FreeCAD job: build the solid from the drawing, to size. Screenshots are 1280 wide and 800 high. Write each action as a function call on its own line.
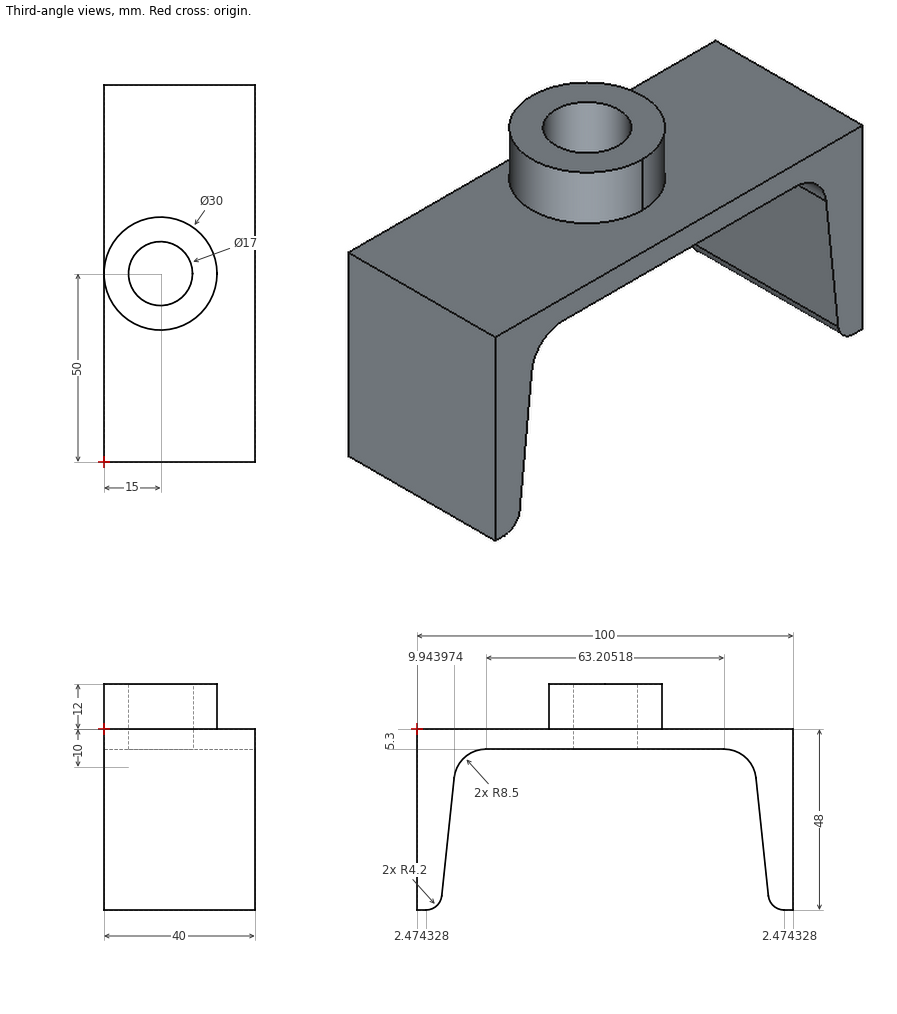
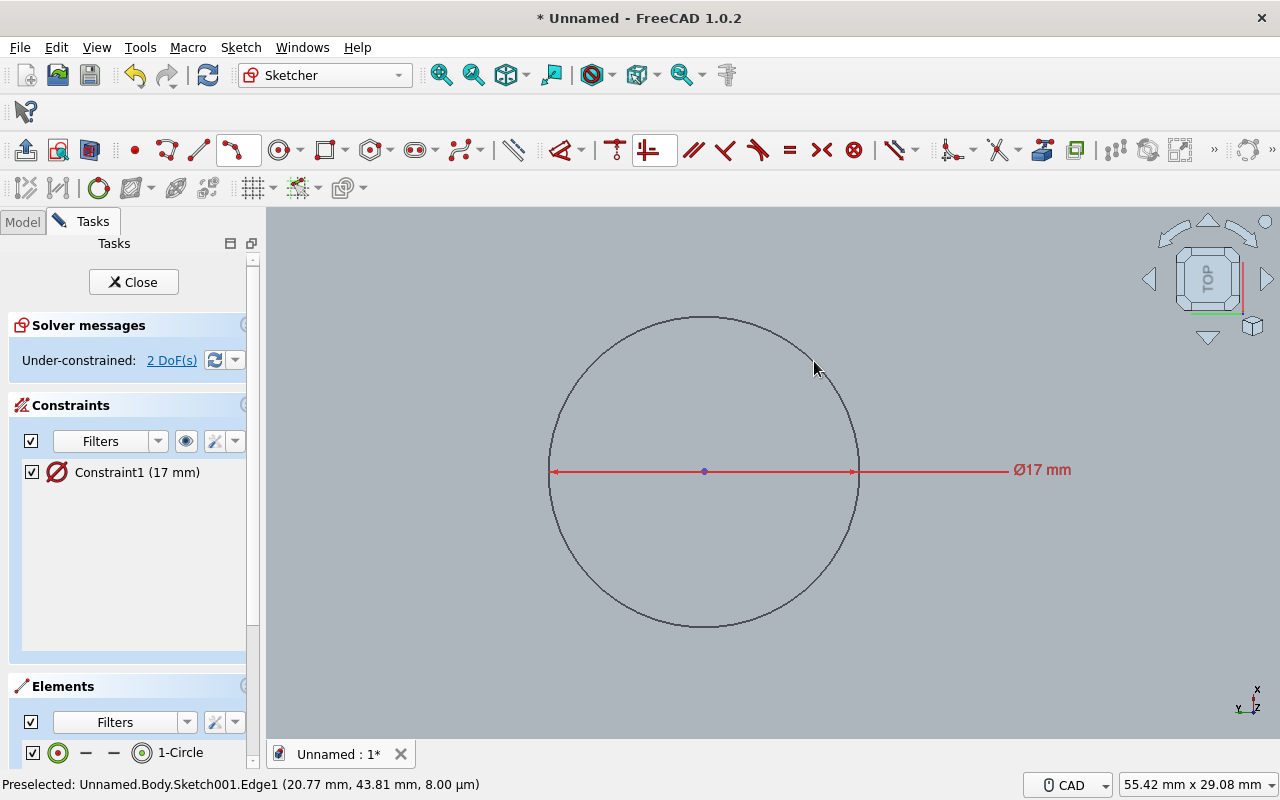
click(560, 150)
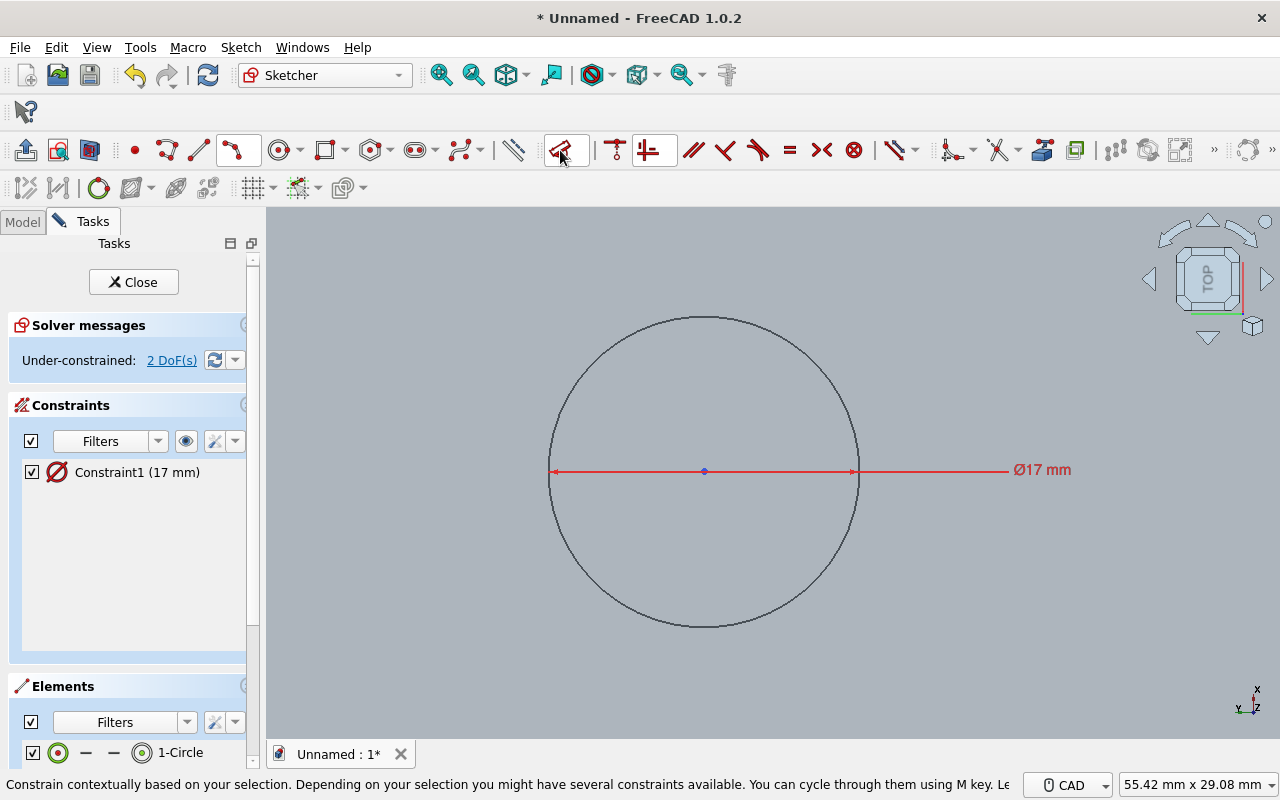
click(704, 472)
click(909, 438)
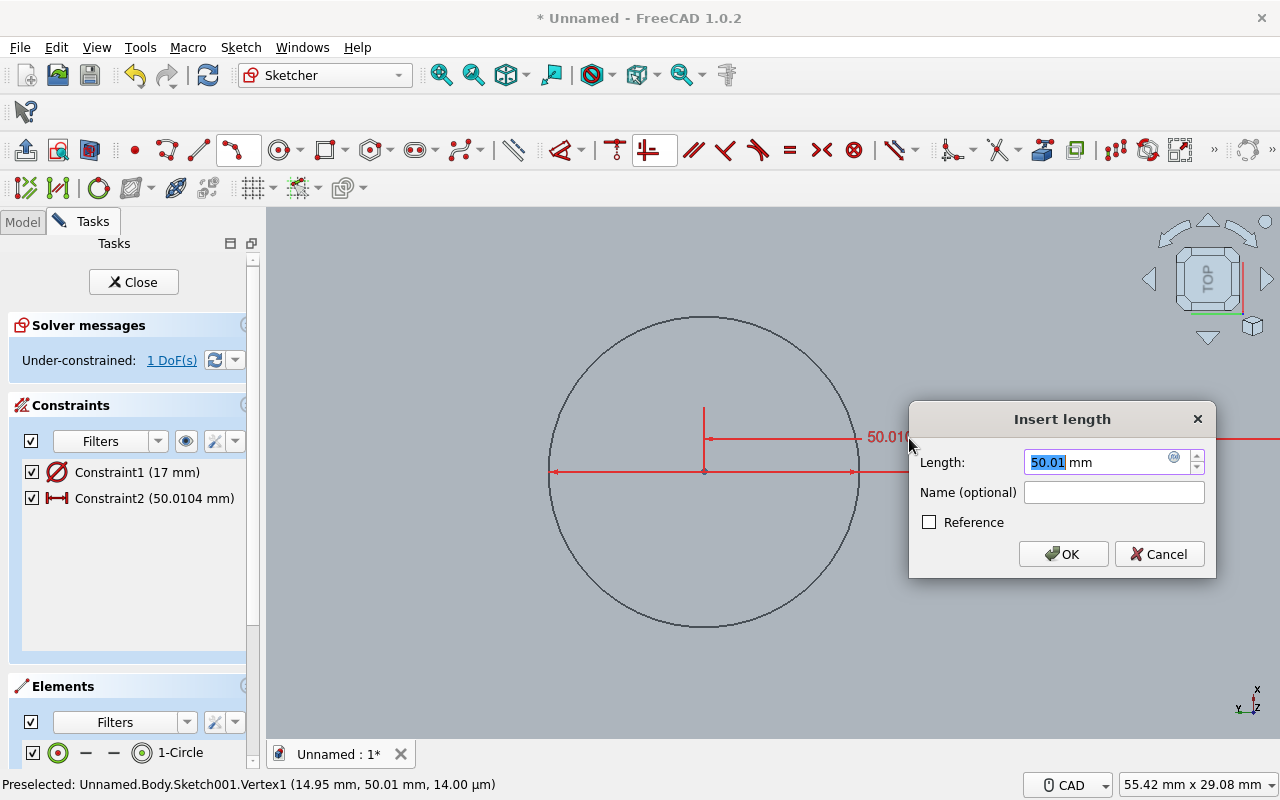
text(50)
key(Return)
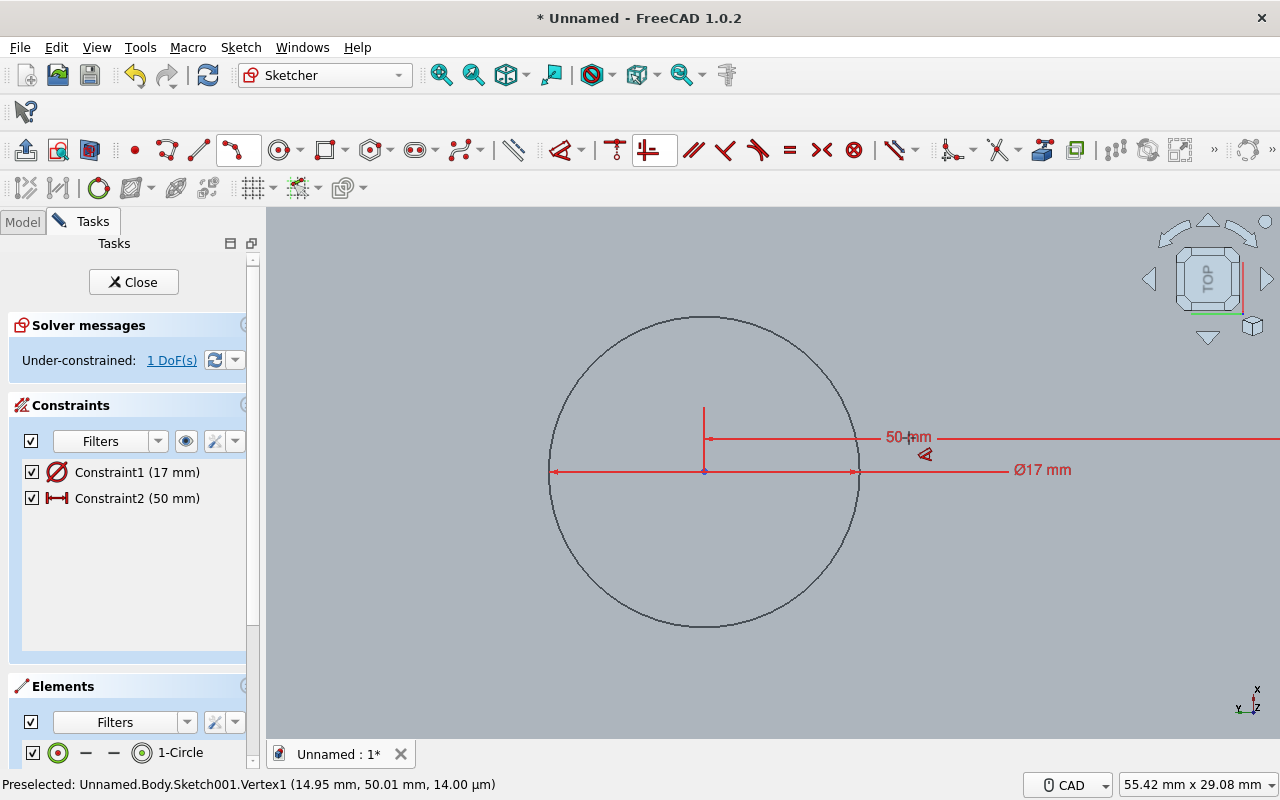
click(704, 472)
click(670, 592)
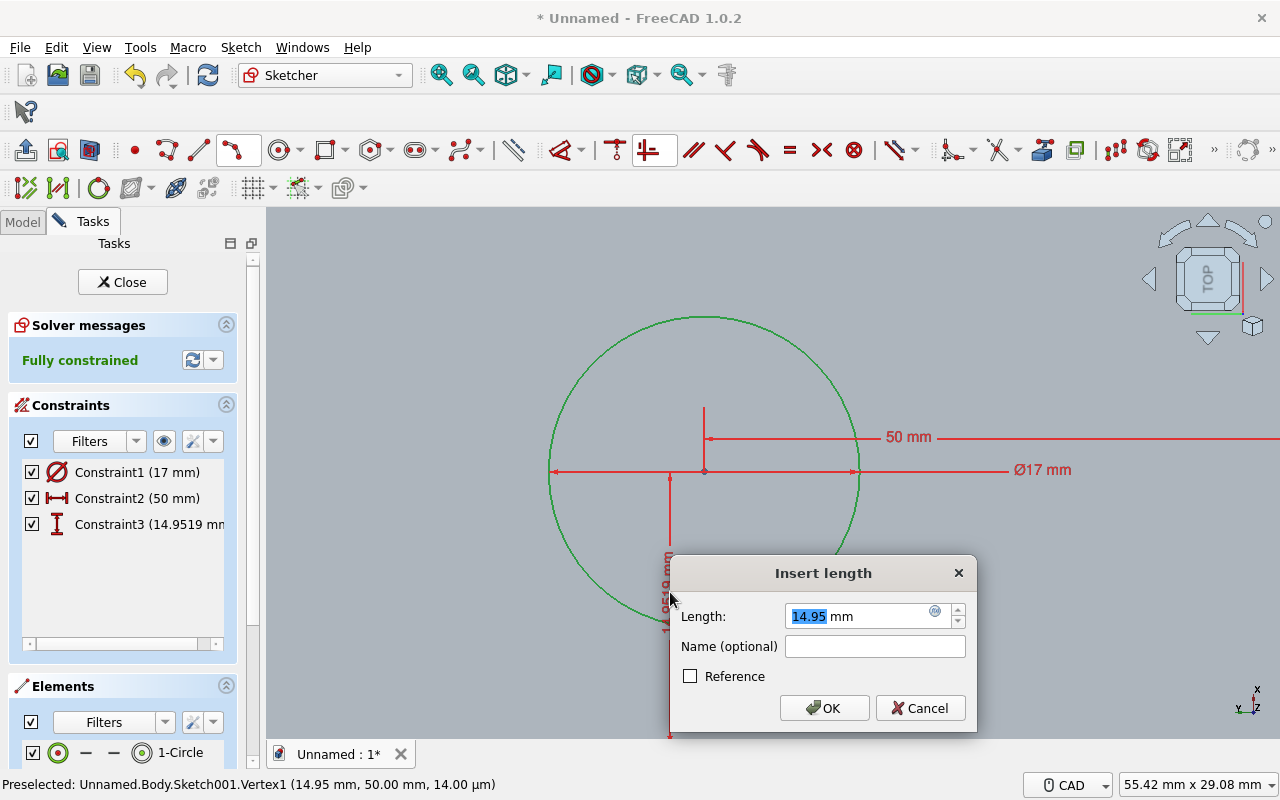
text(15)
key(Return)
key(Escape)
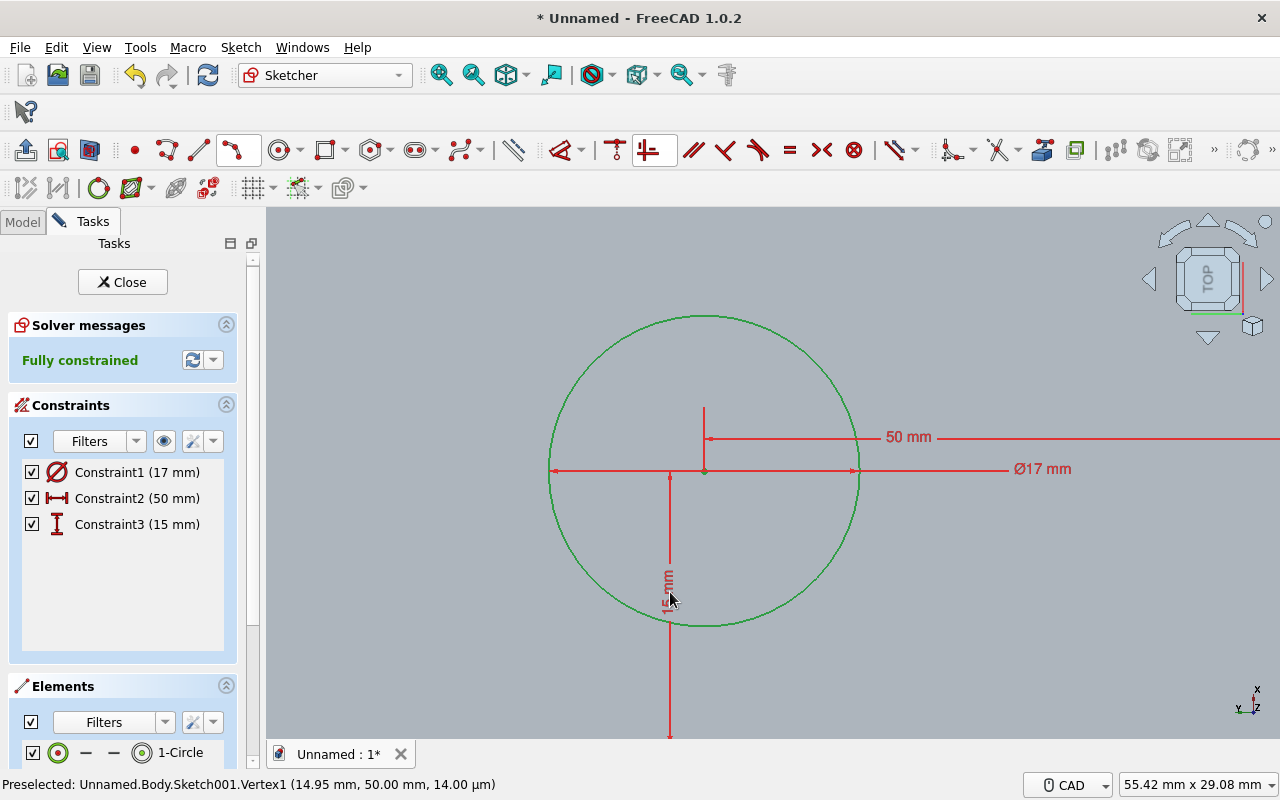
click(123, 282)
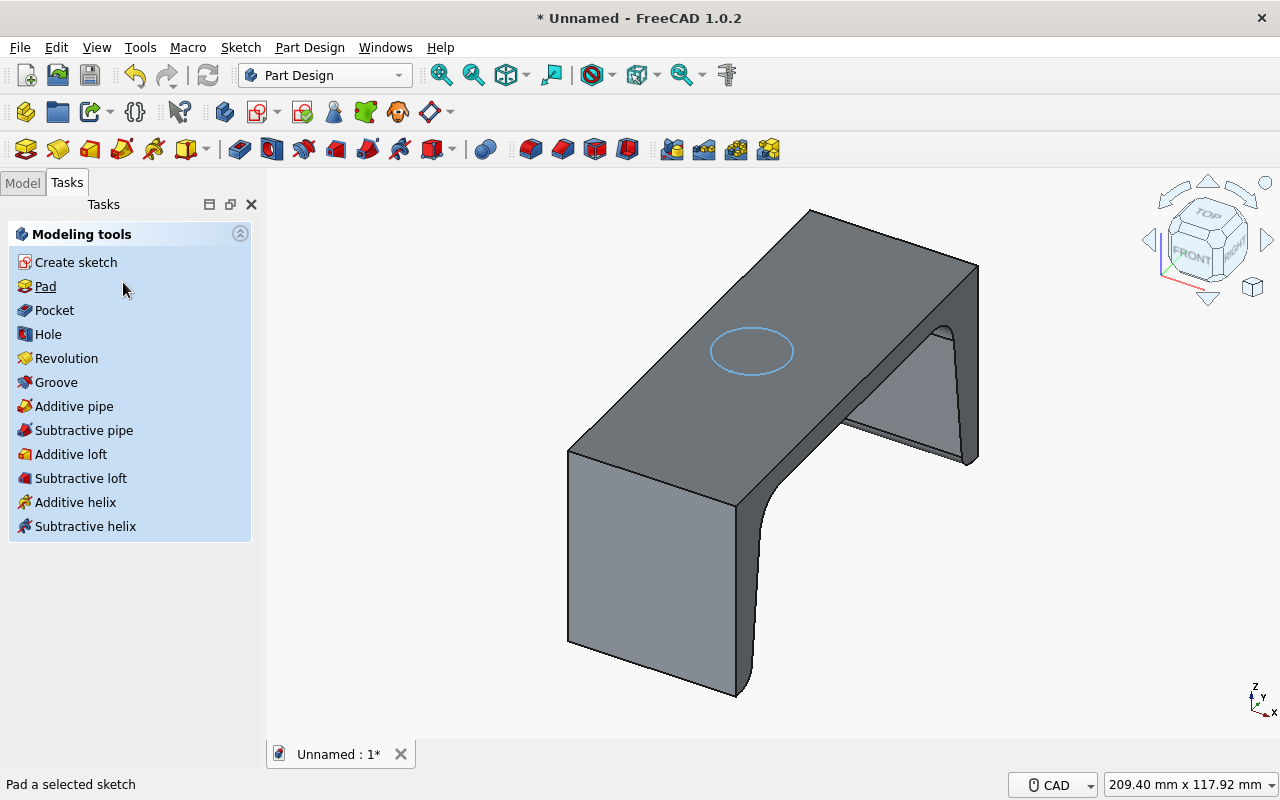
click(240, 150)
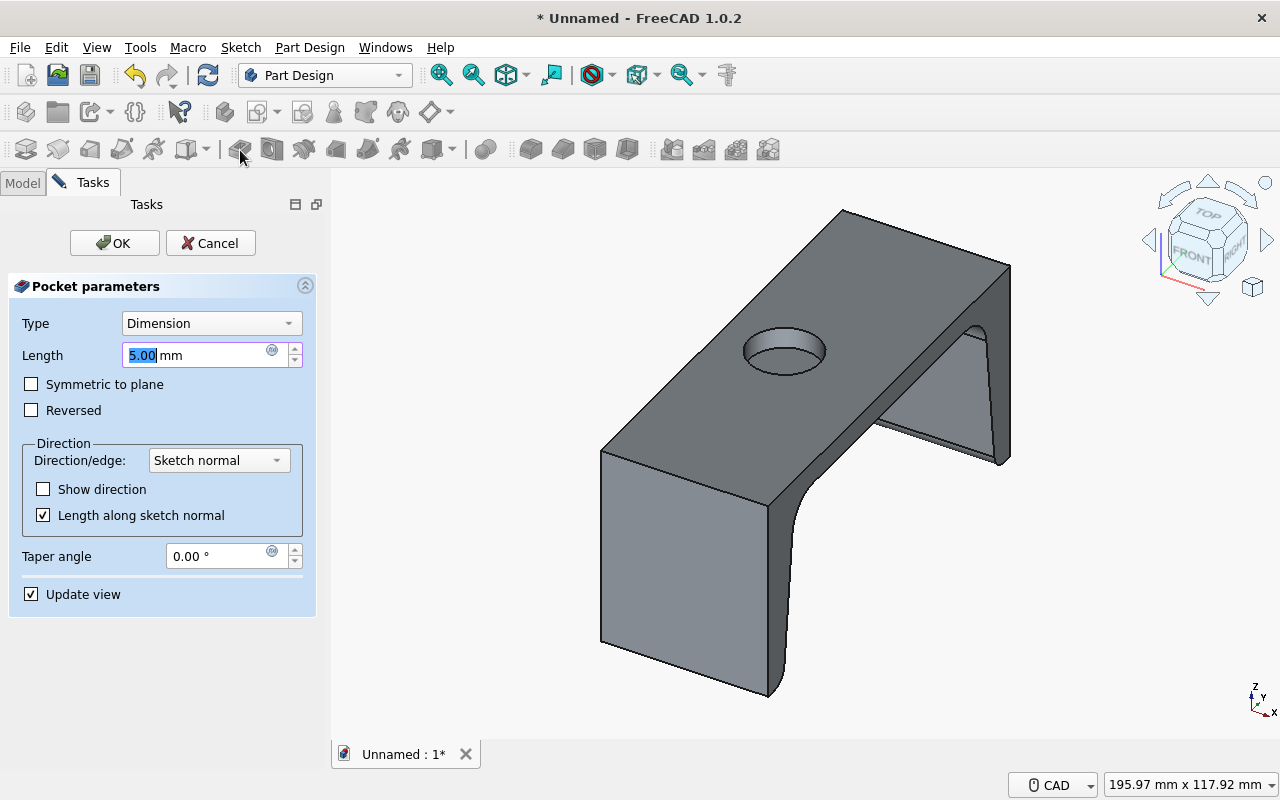
text(10)
key(Tab)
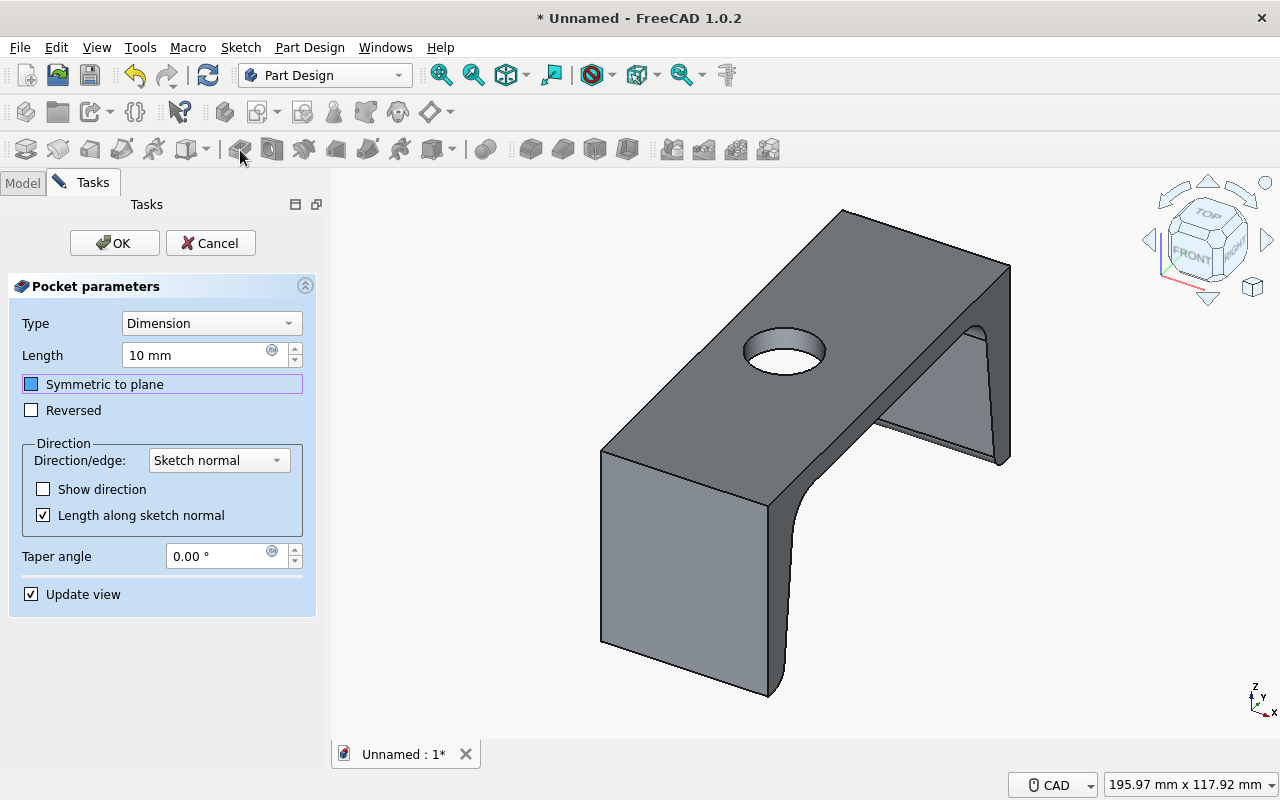
click(115, 243)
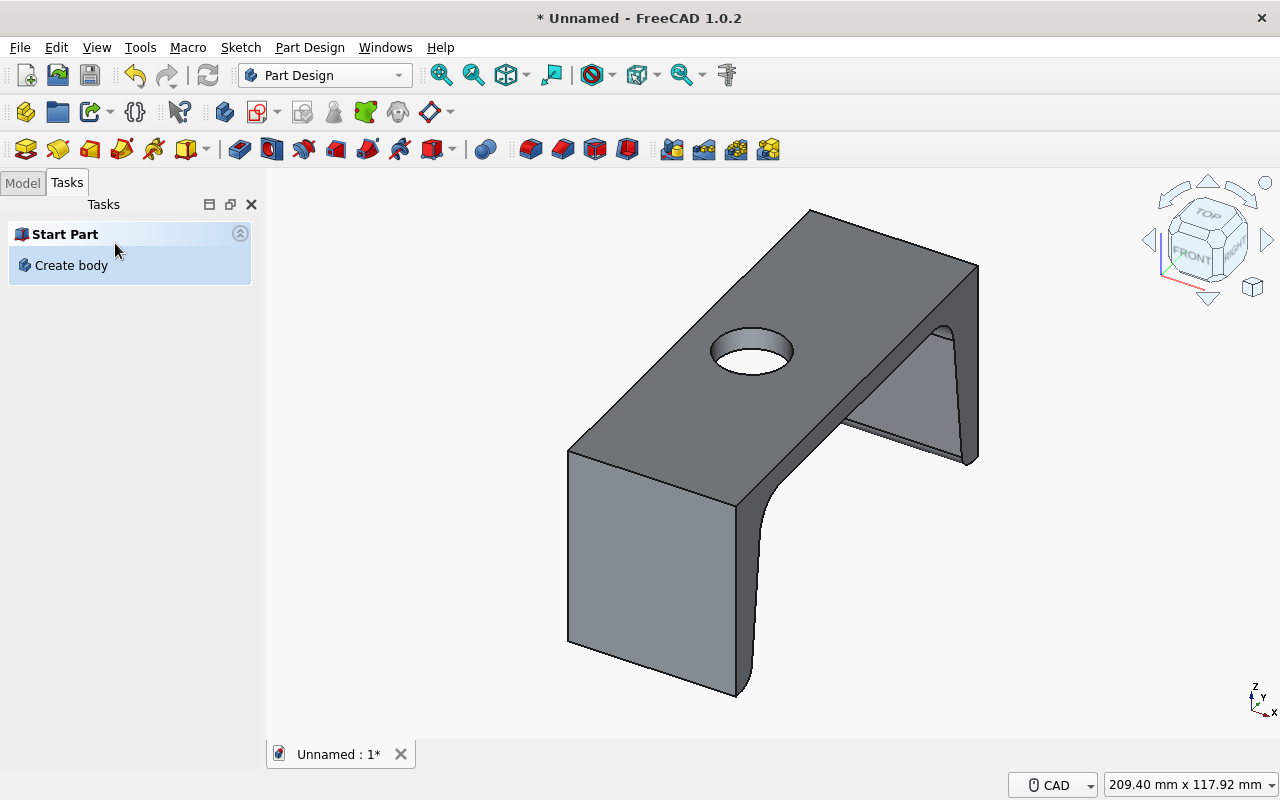
click(226, 112)